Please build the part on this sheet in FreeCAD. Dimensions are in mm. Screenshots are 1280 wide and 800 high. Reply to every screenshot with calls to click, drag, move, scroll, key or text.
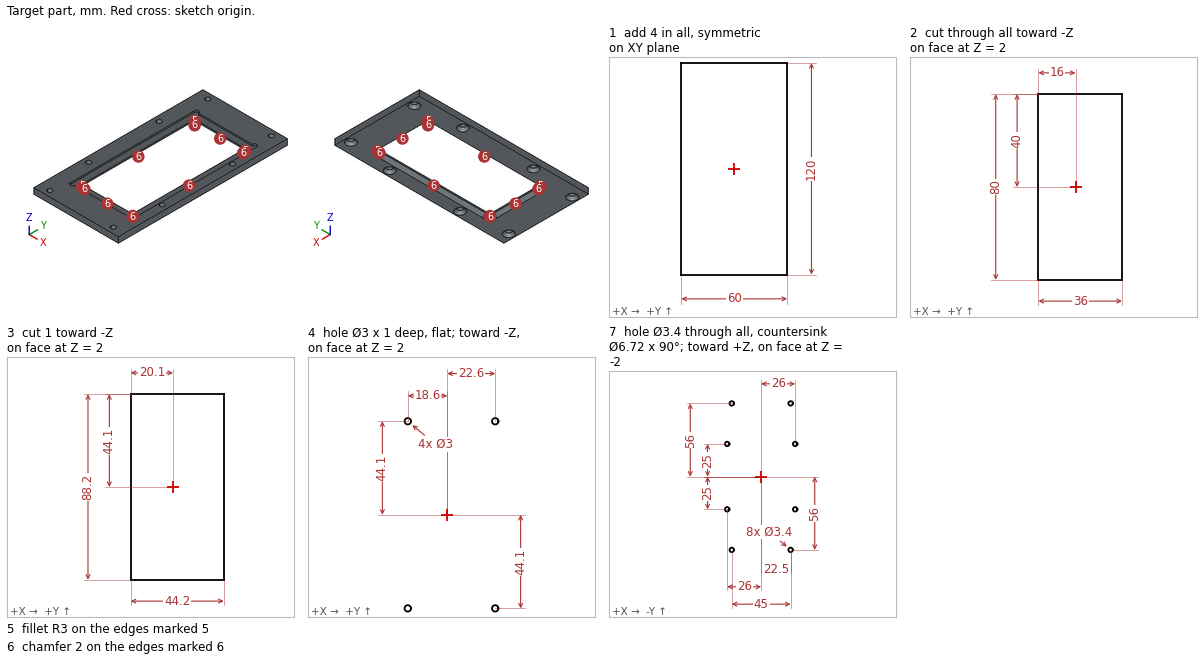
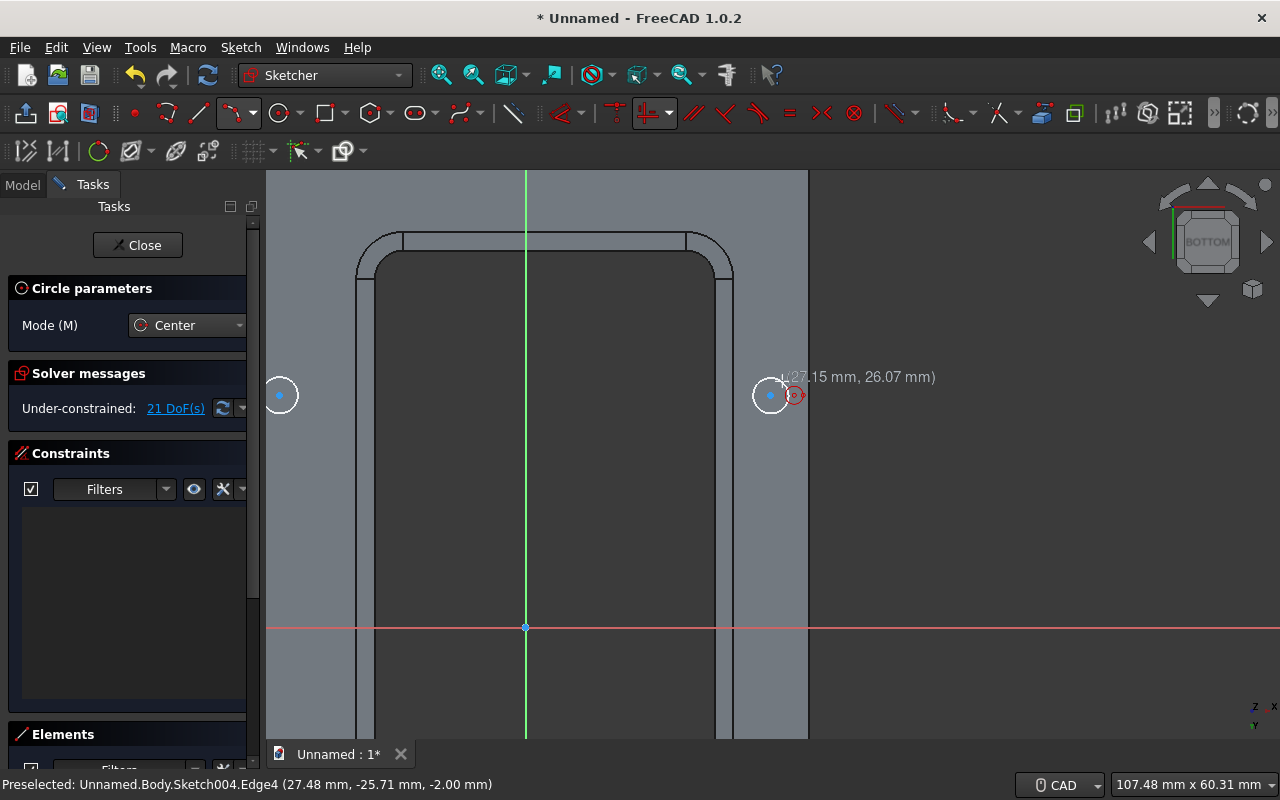
scroll(782, 380, down, 6)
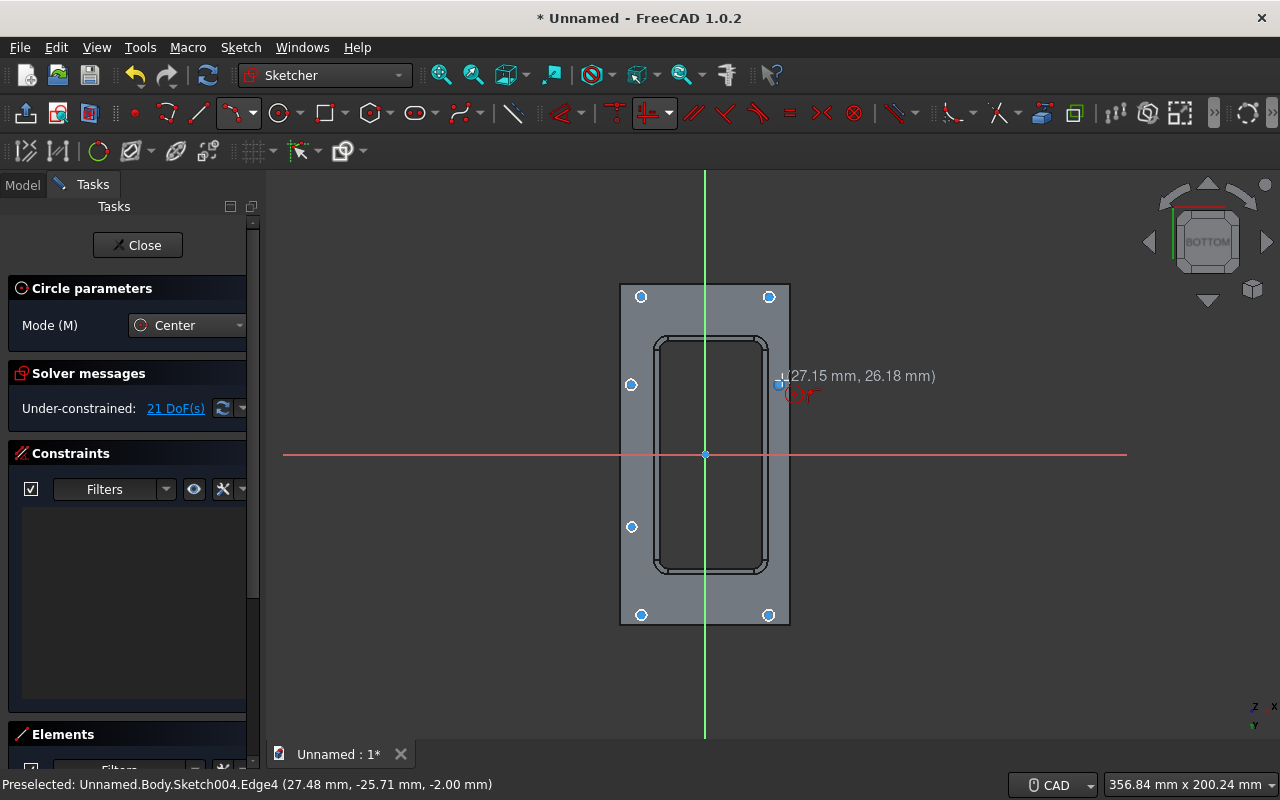
scroll(779, 526, up, 8)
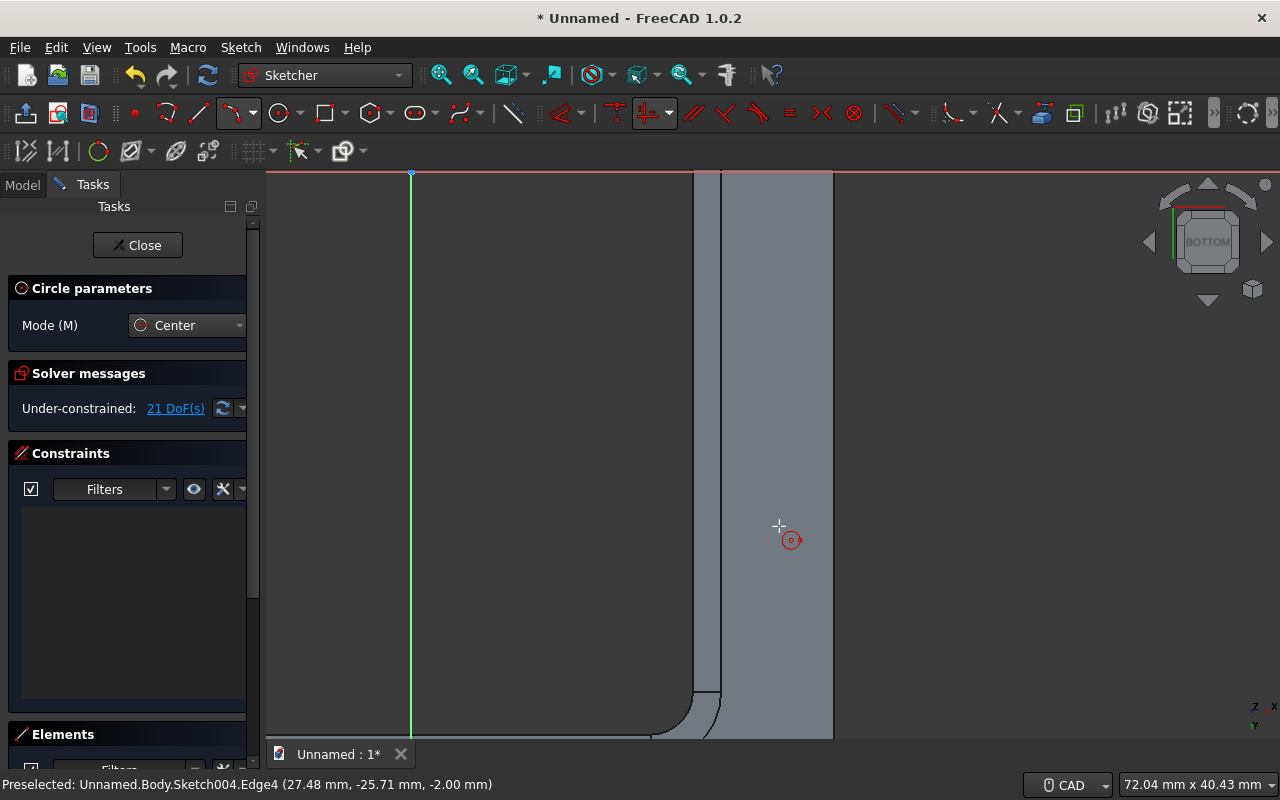
scroll(779, 526, down, 8)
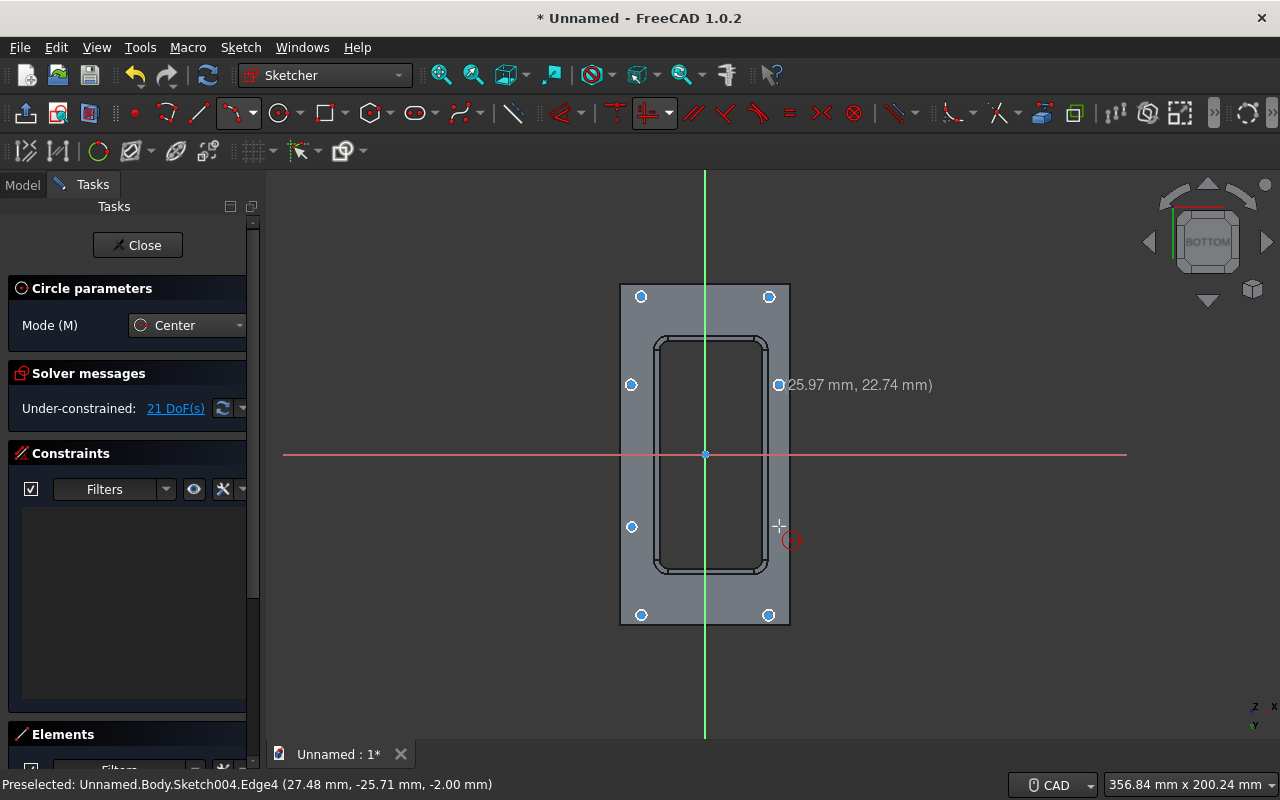
click(779, 526)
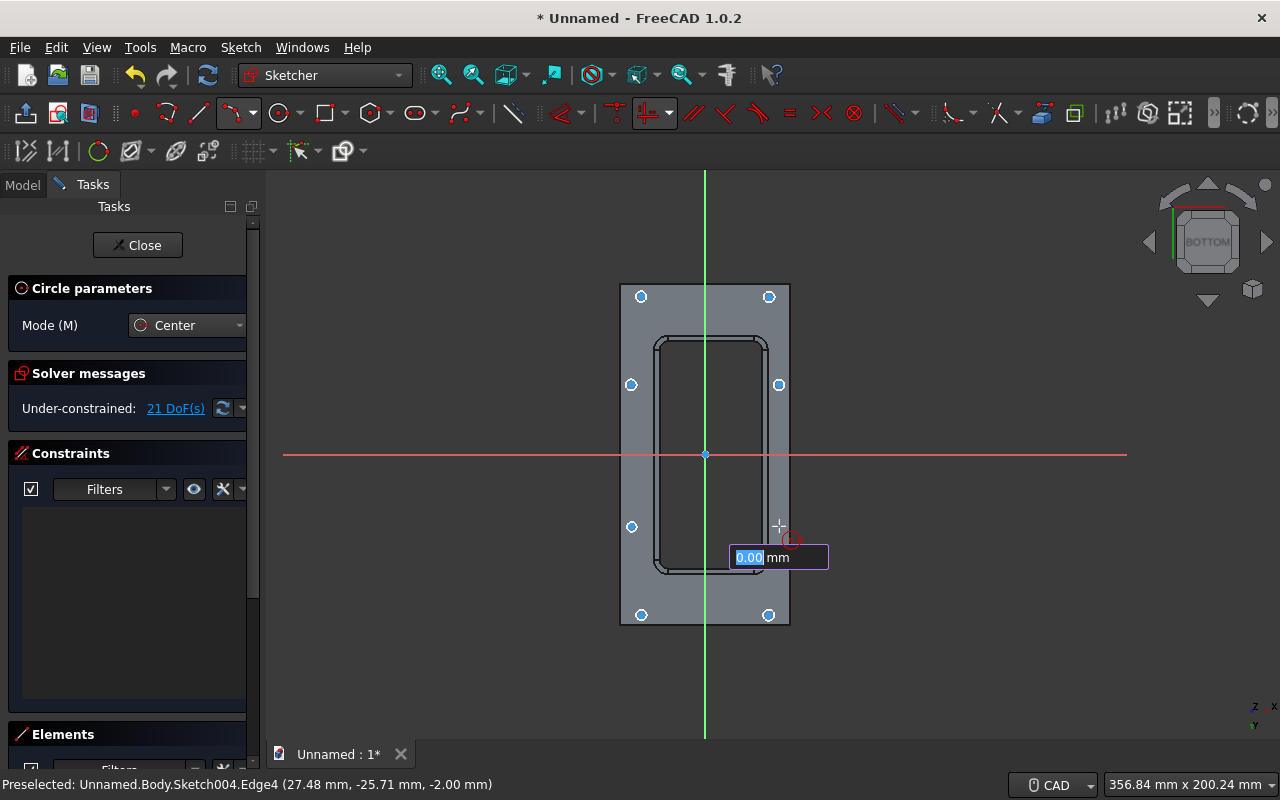
scroll(782, 523, up, 6)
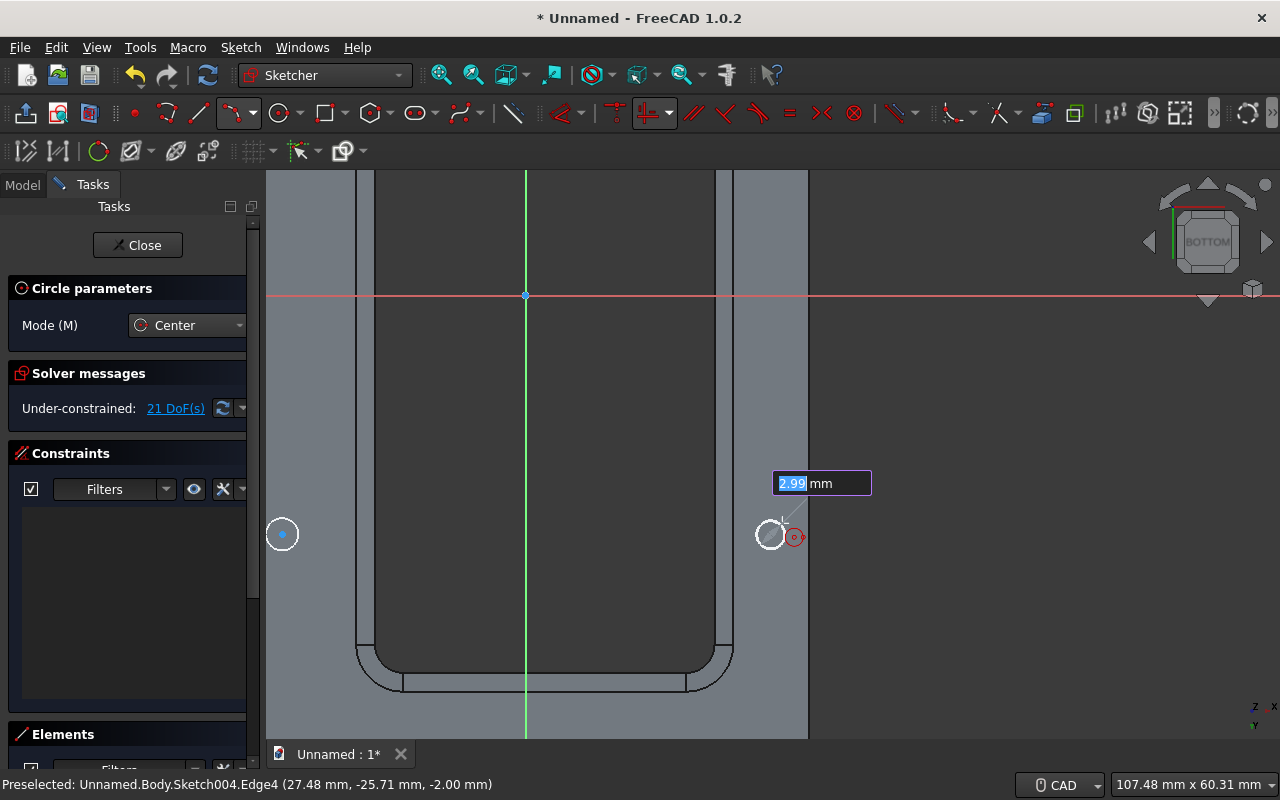
click(782, 520)
key(Escape)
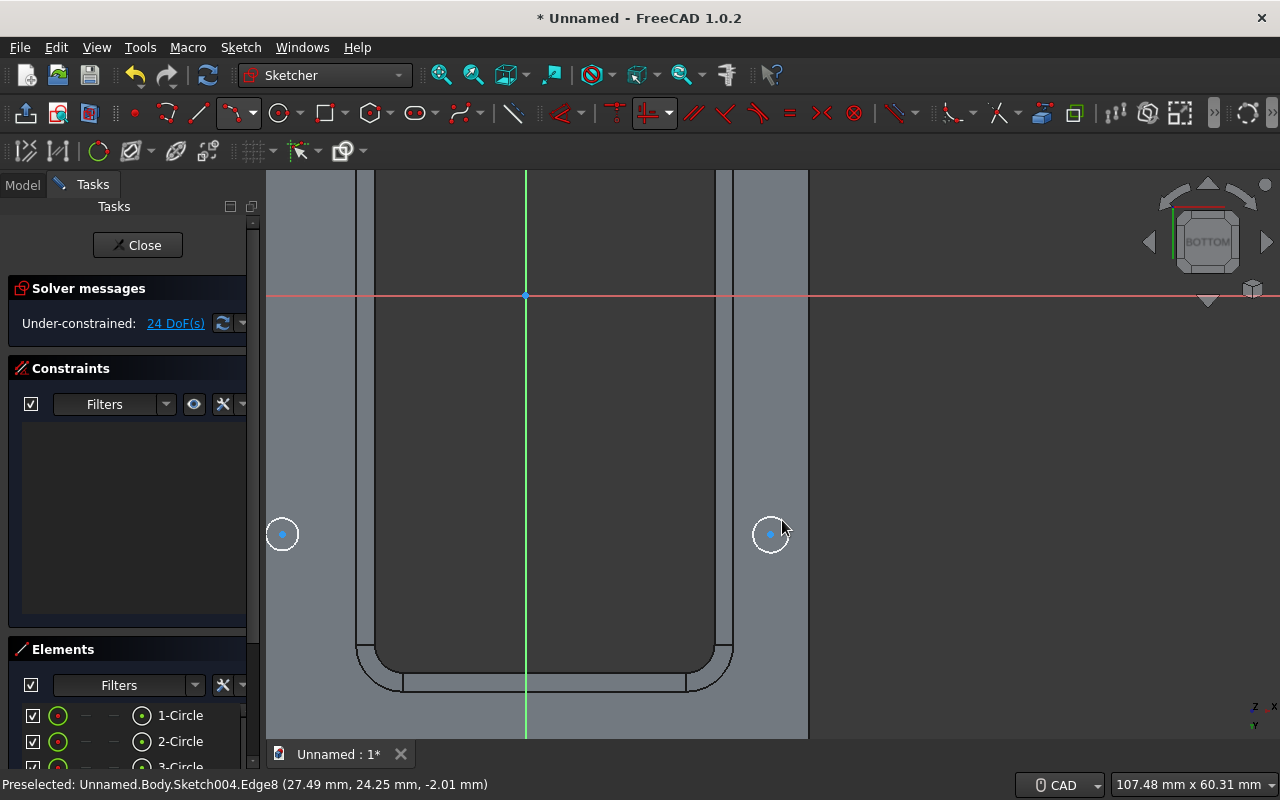
scroll(782, 523, down, 6)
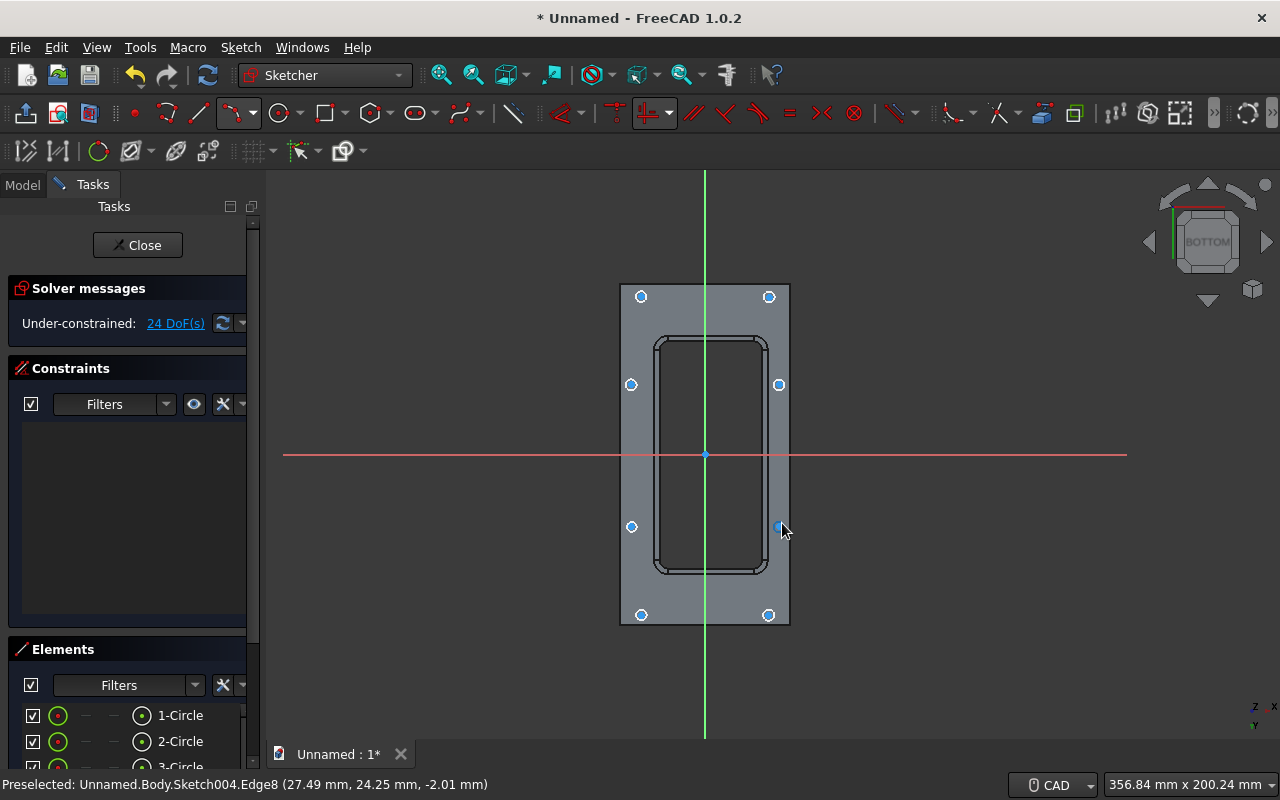
scroll(773, 611, up, 5)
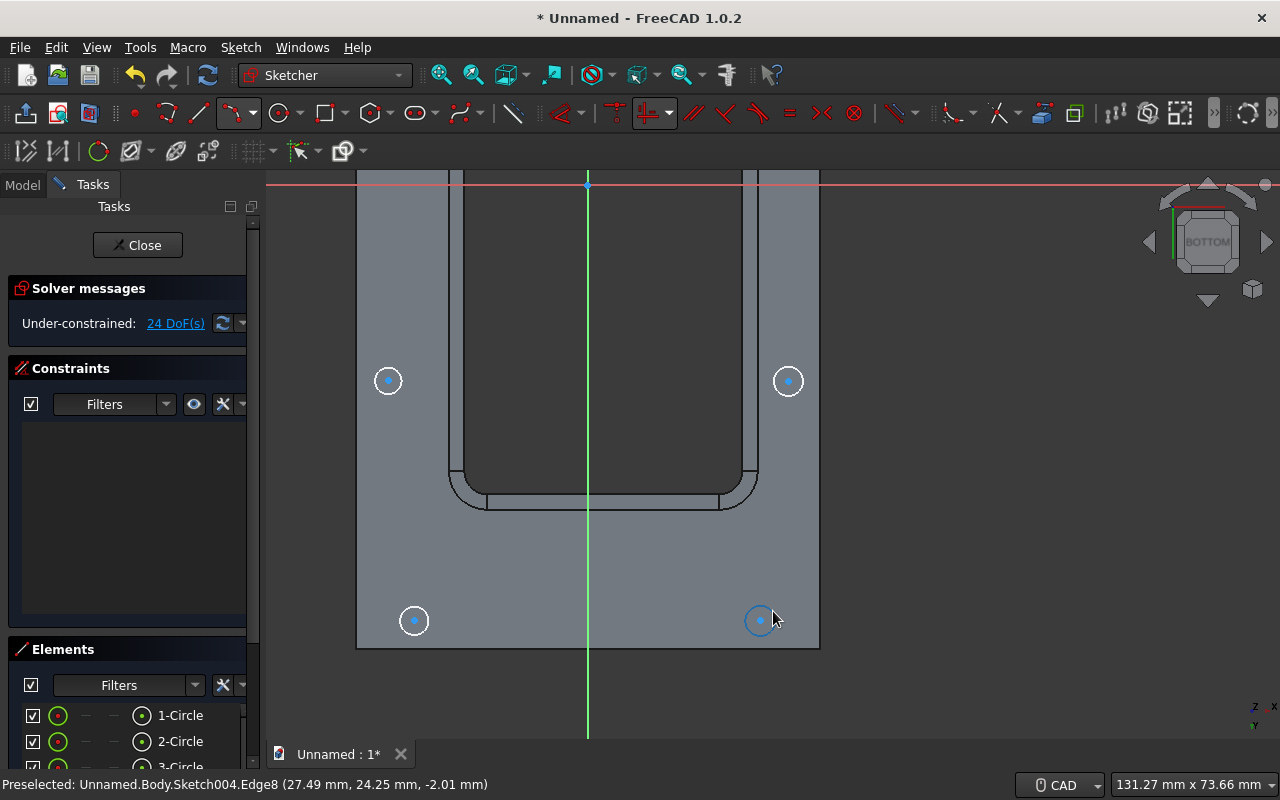
click(771, 610)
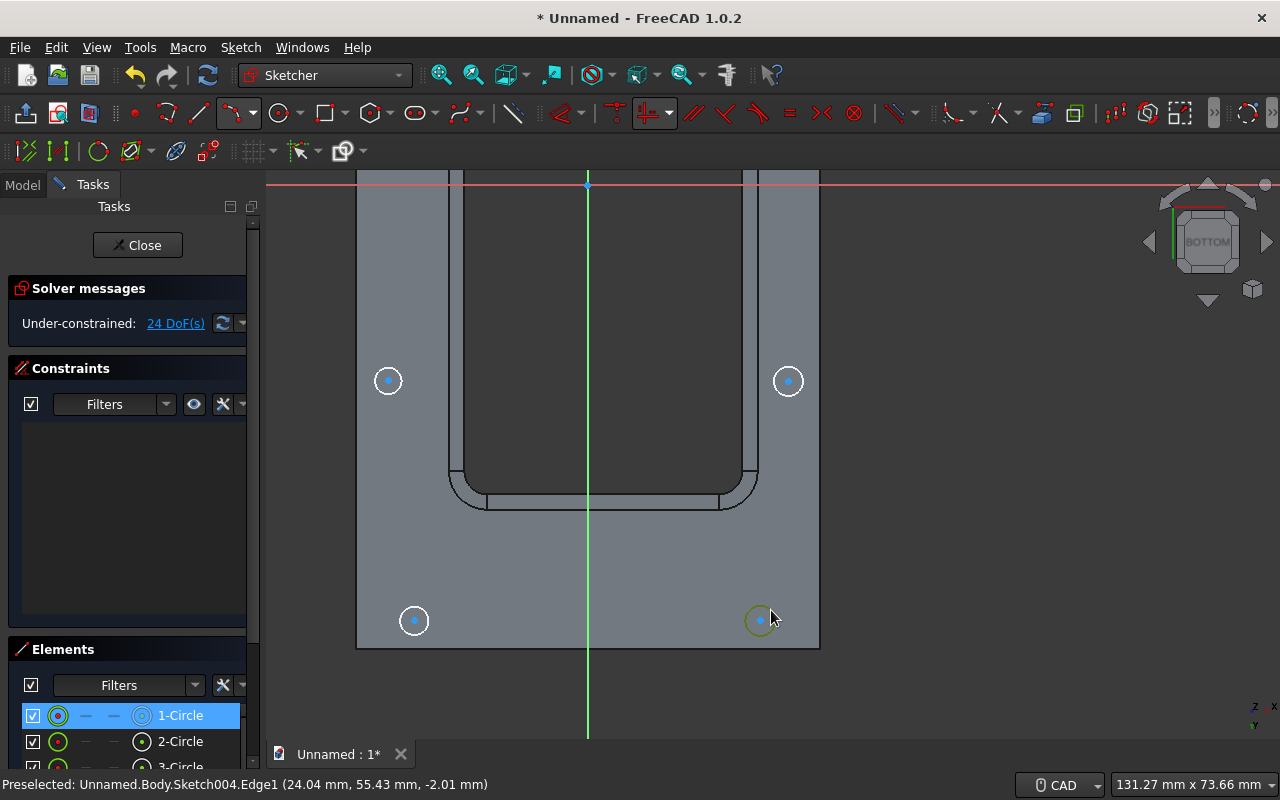
click(424, 611)